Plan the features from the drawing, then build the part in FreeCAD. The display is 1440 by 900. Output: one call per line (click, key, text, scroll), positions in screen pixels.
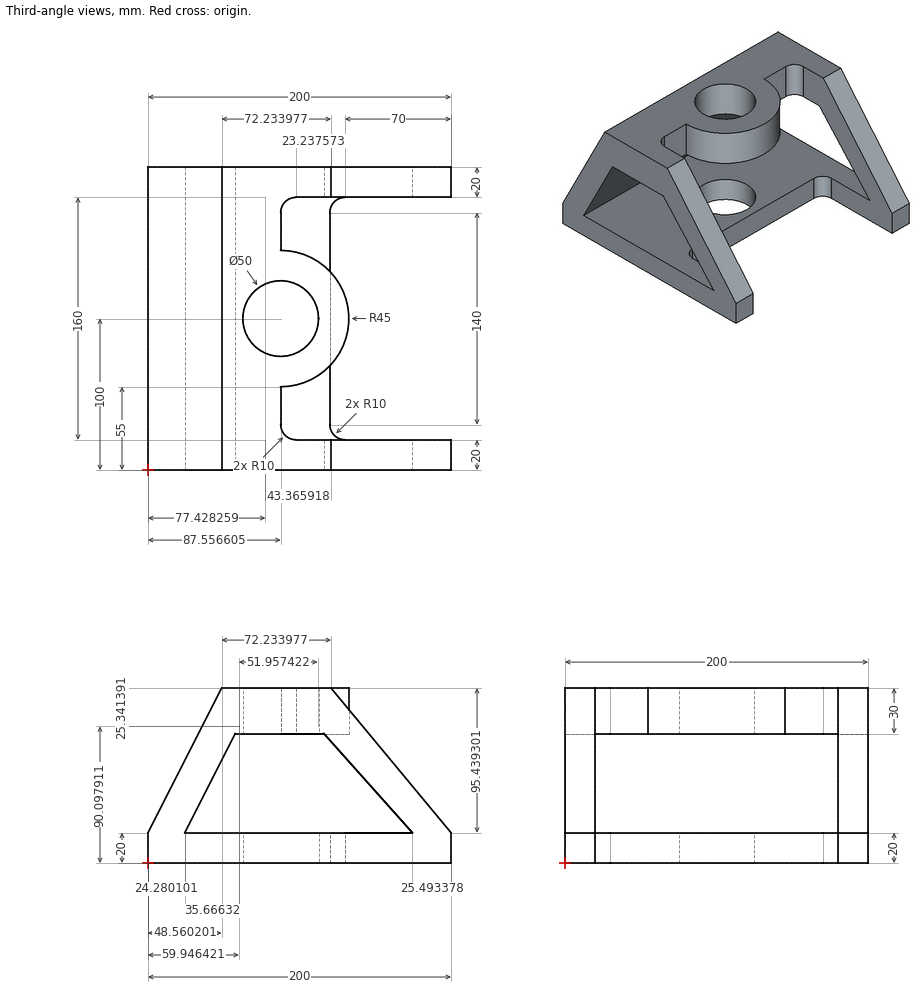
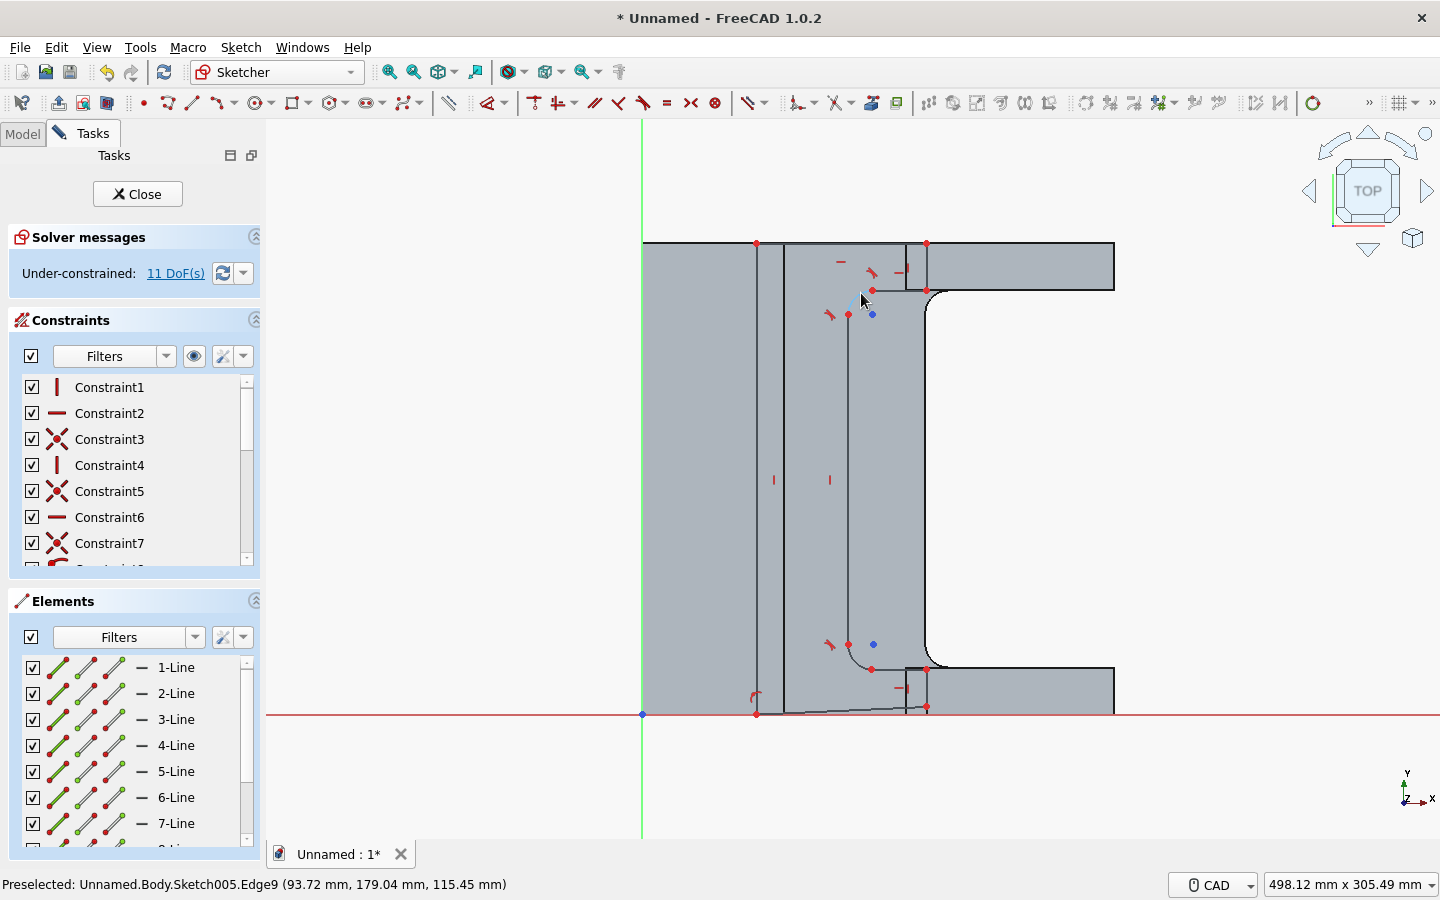
click(910, 670)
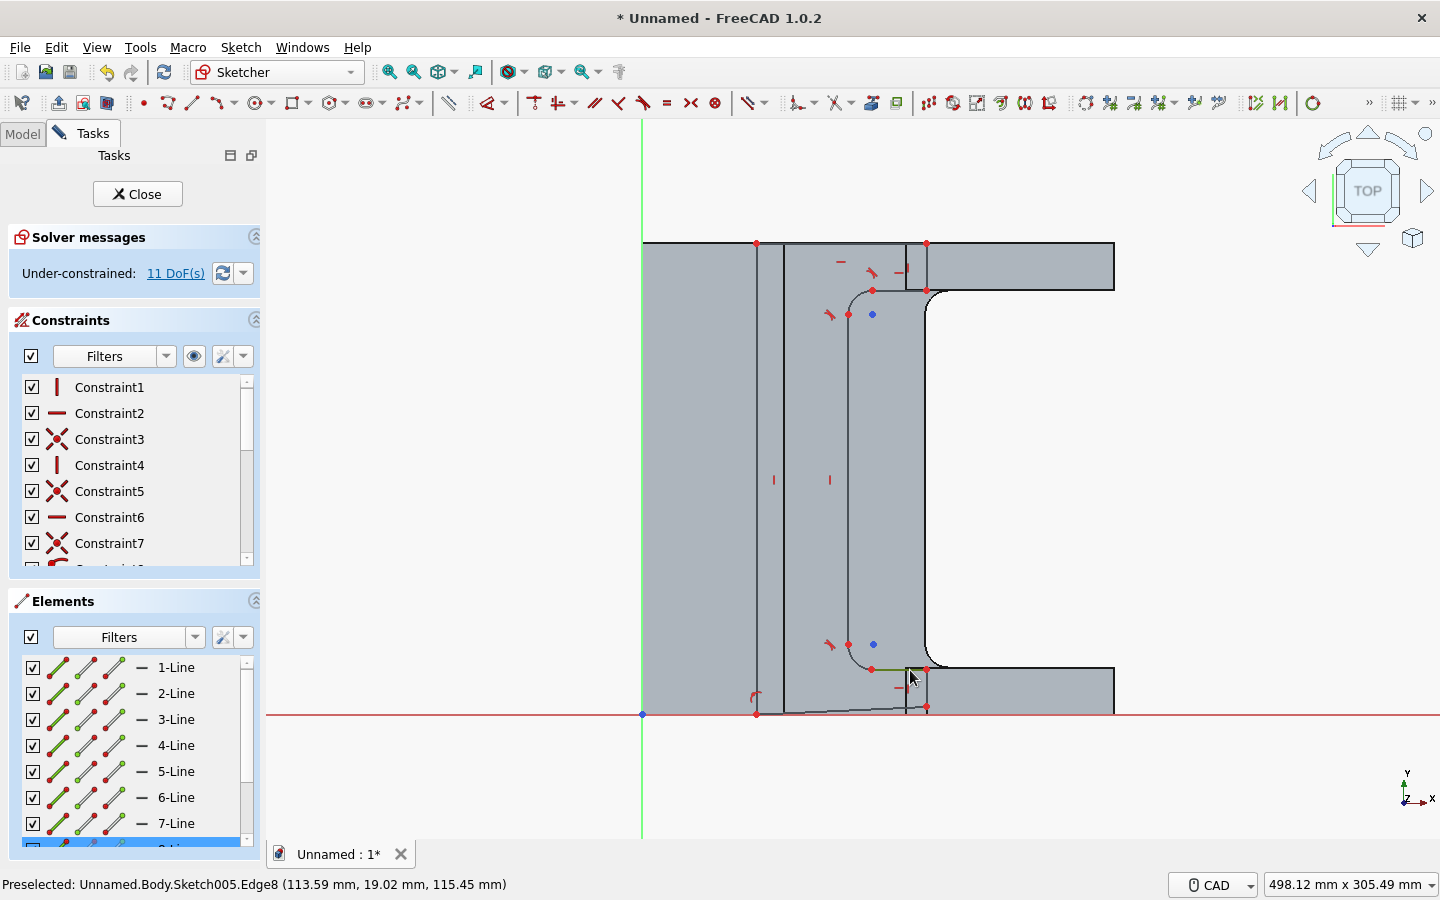
click(851, 655)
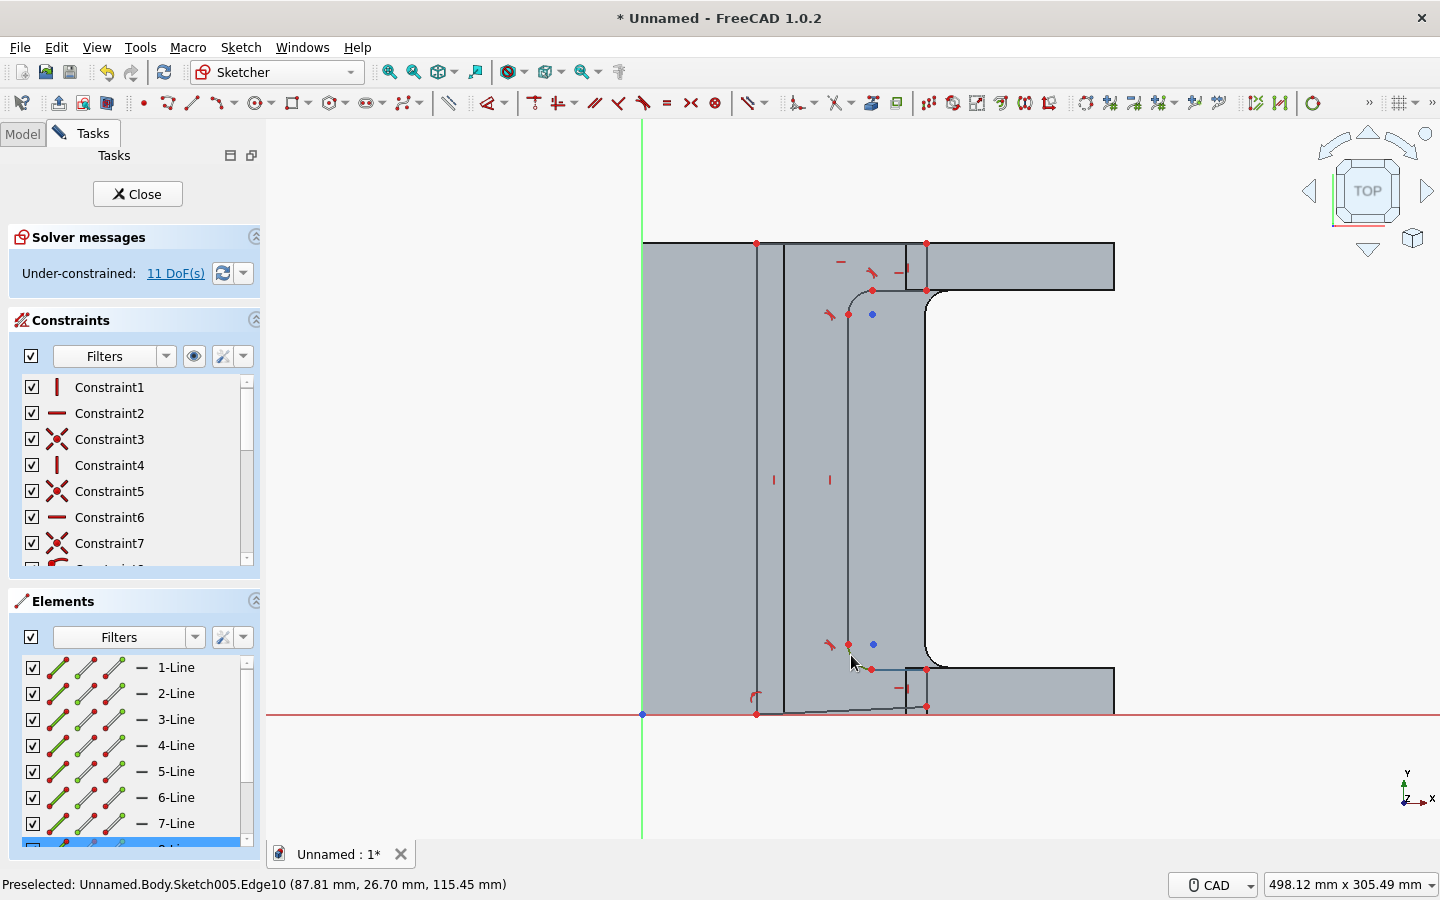
key(t)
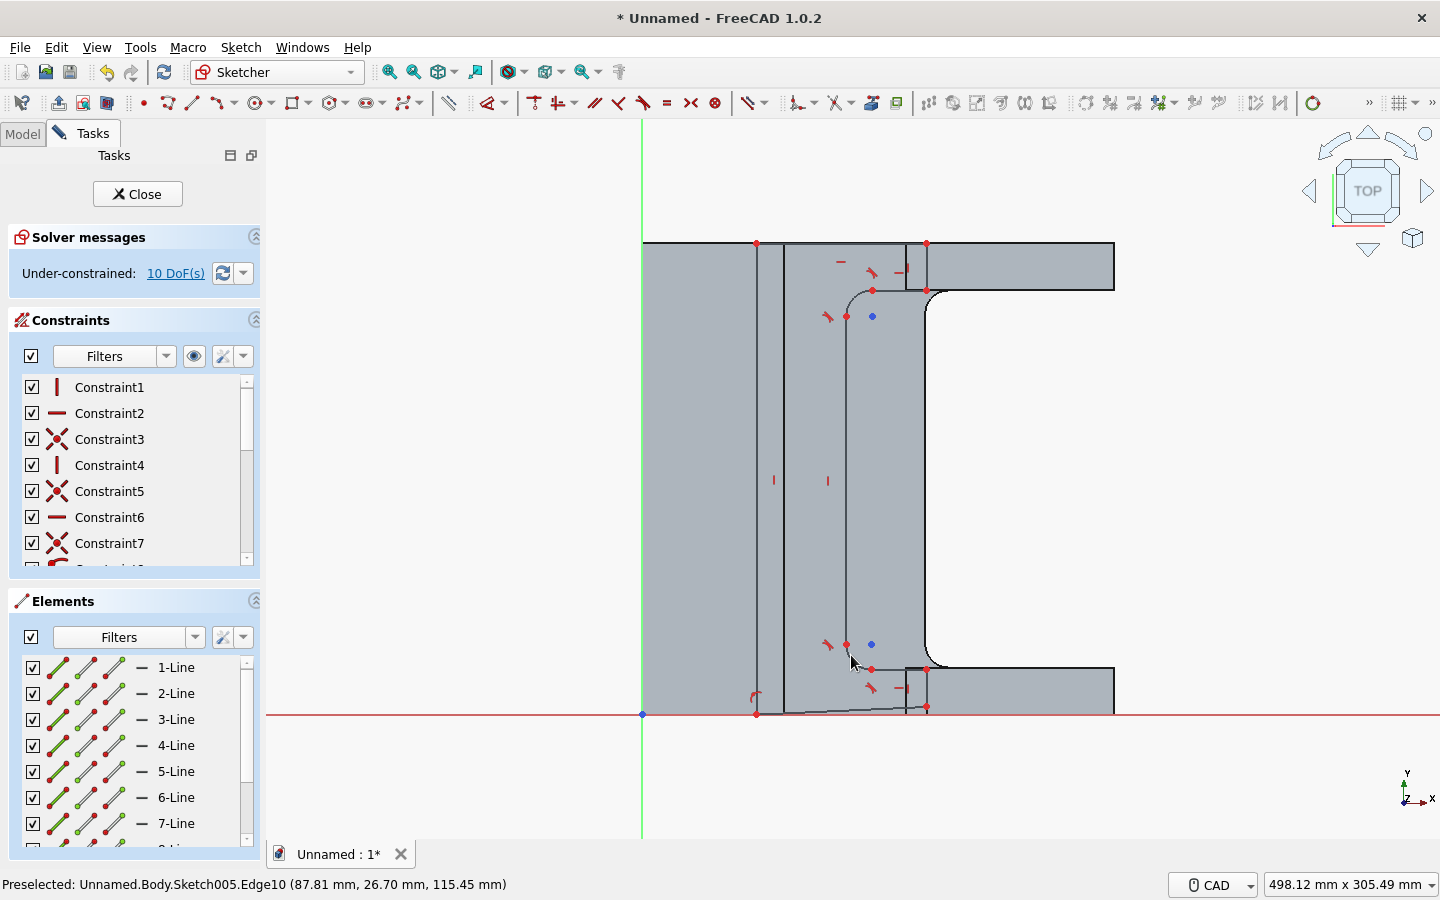
click(808, 712)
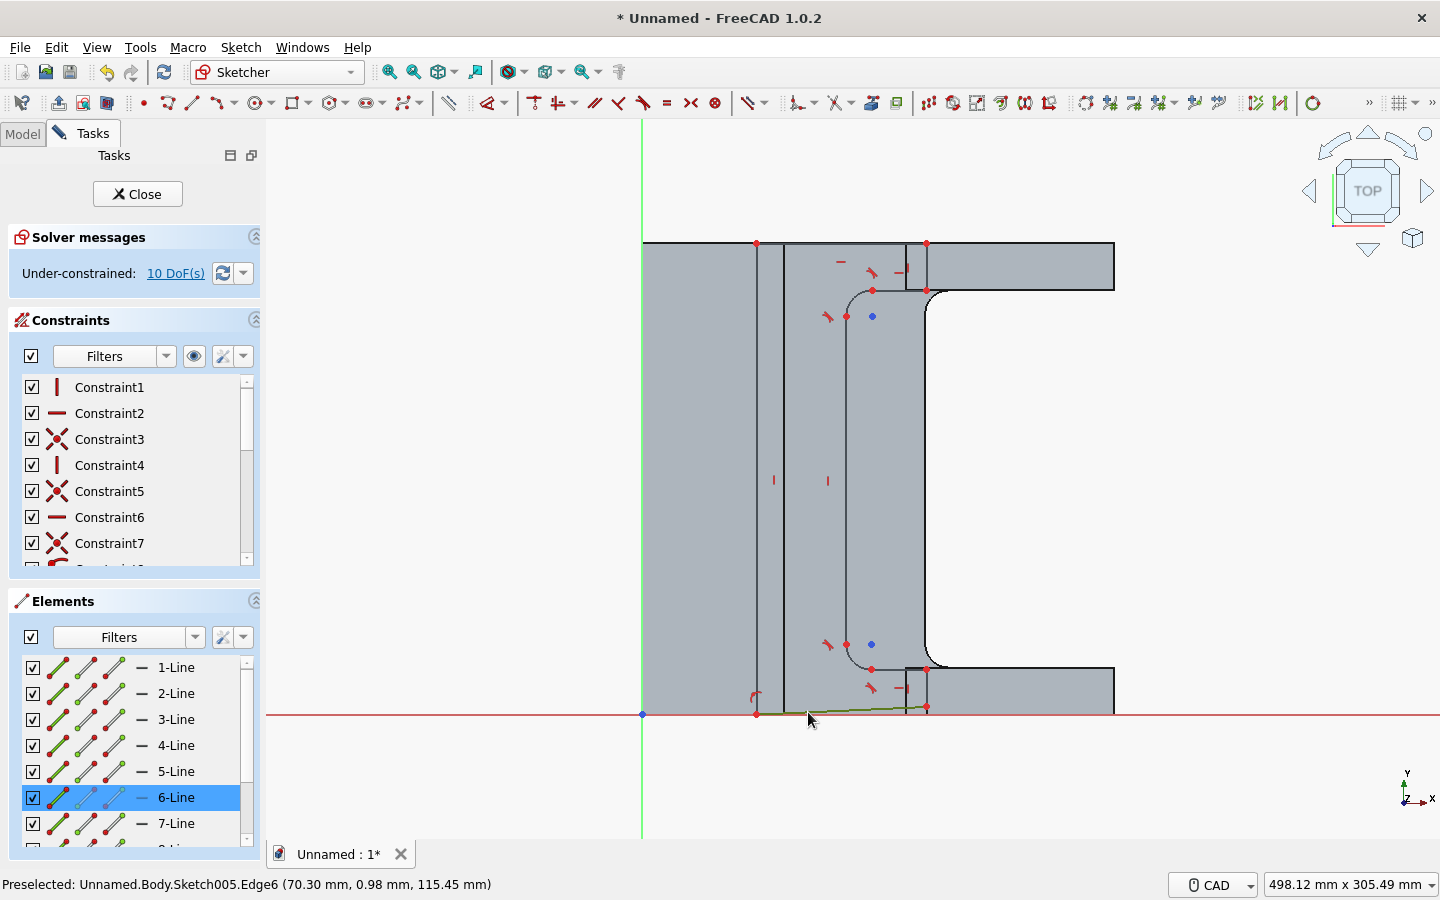
key(h)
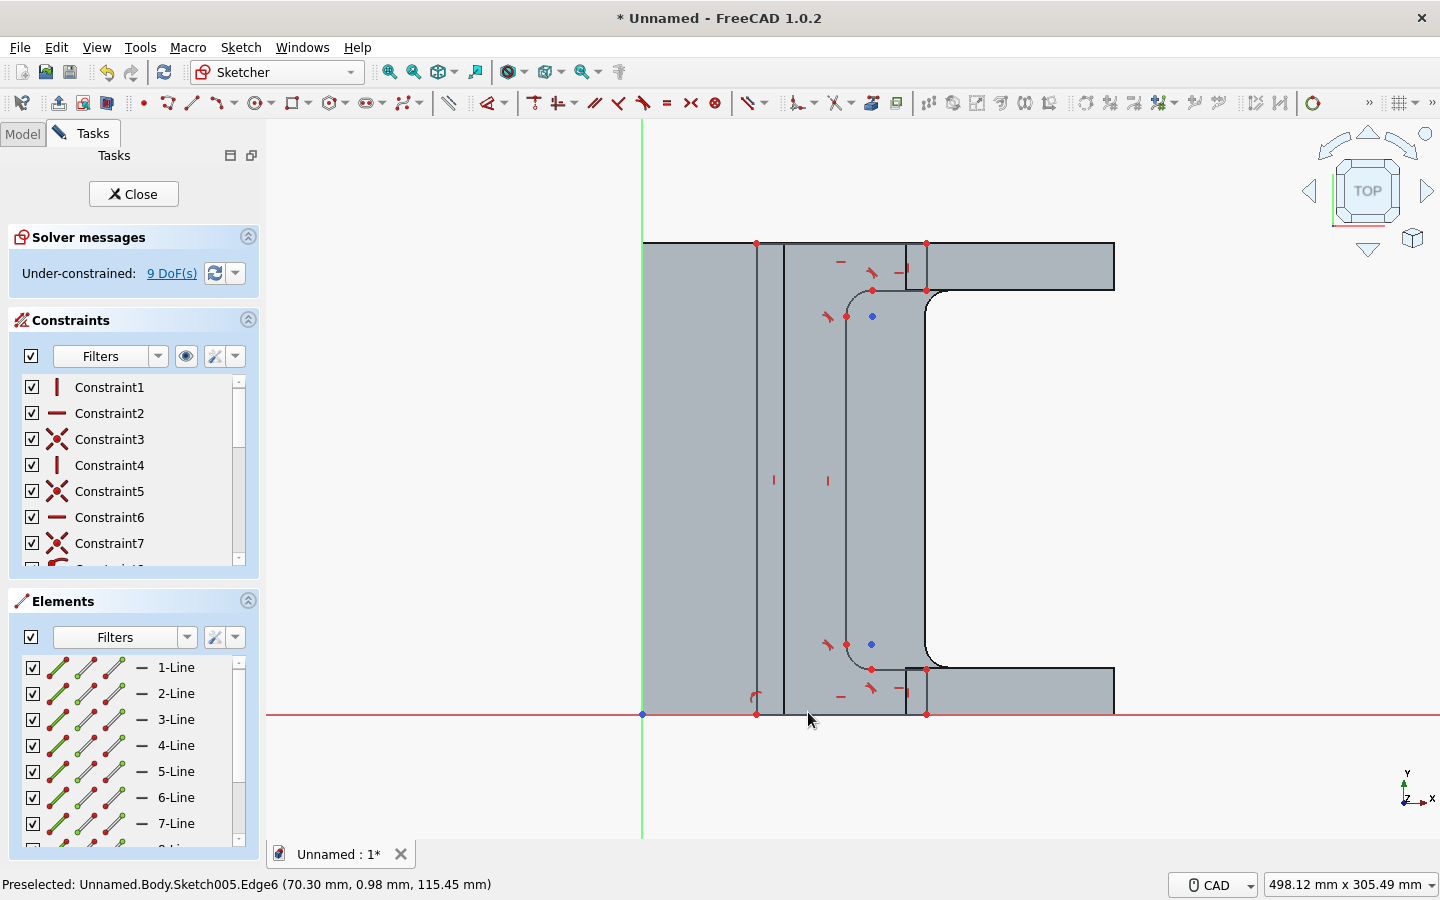
click(860, 293)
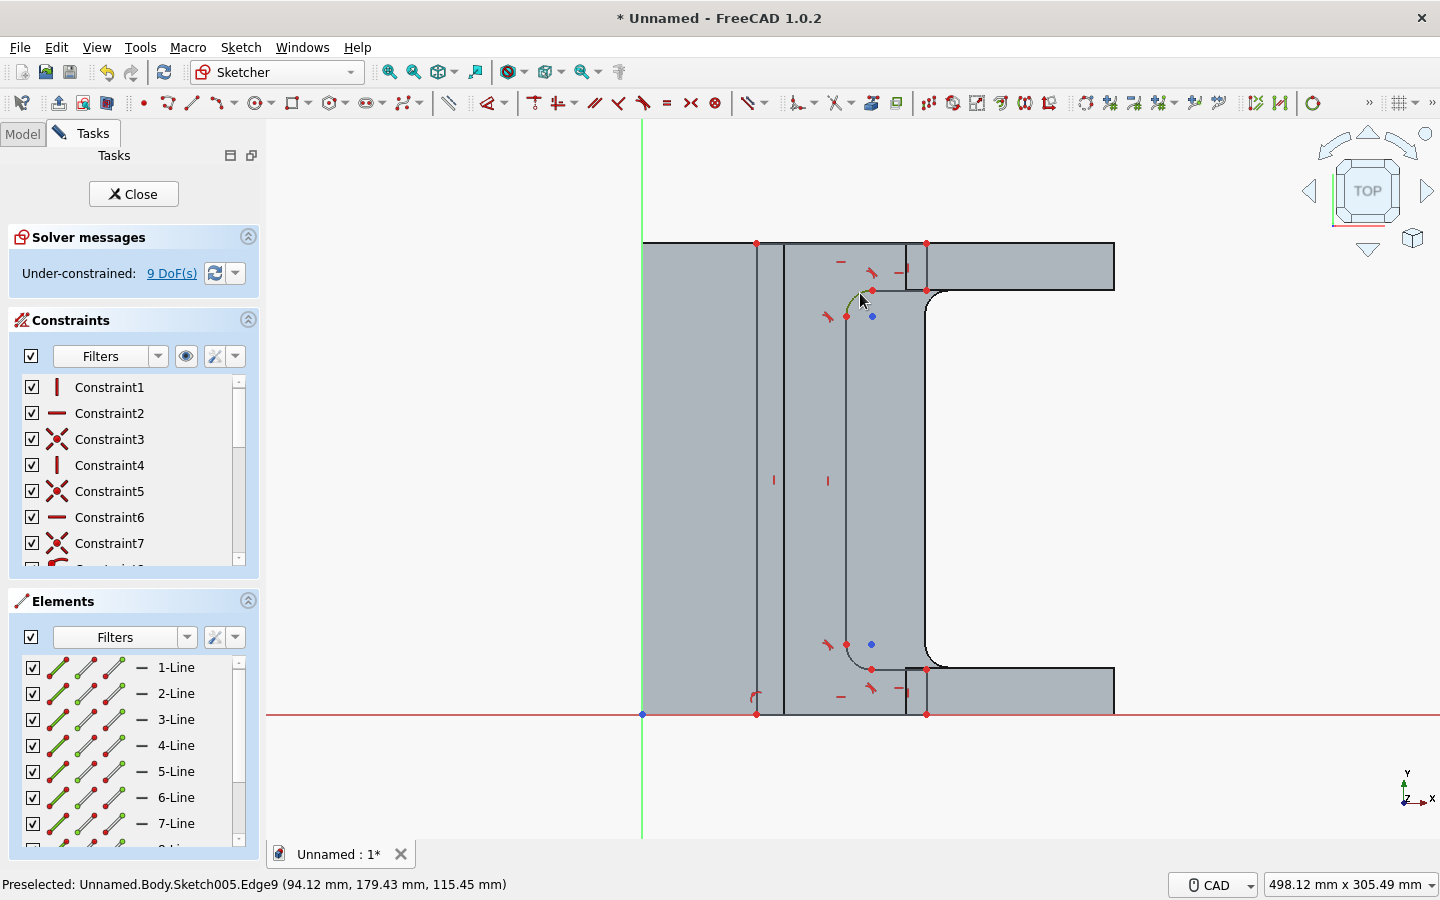
click(849, 656)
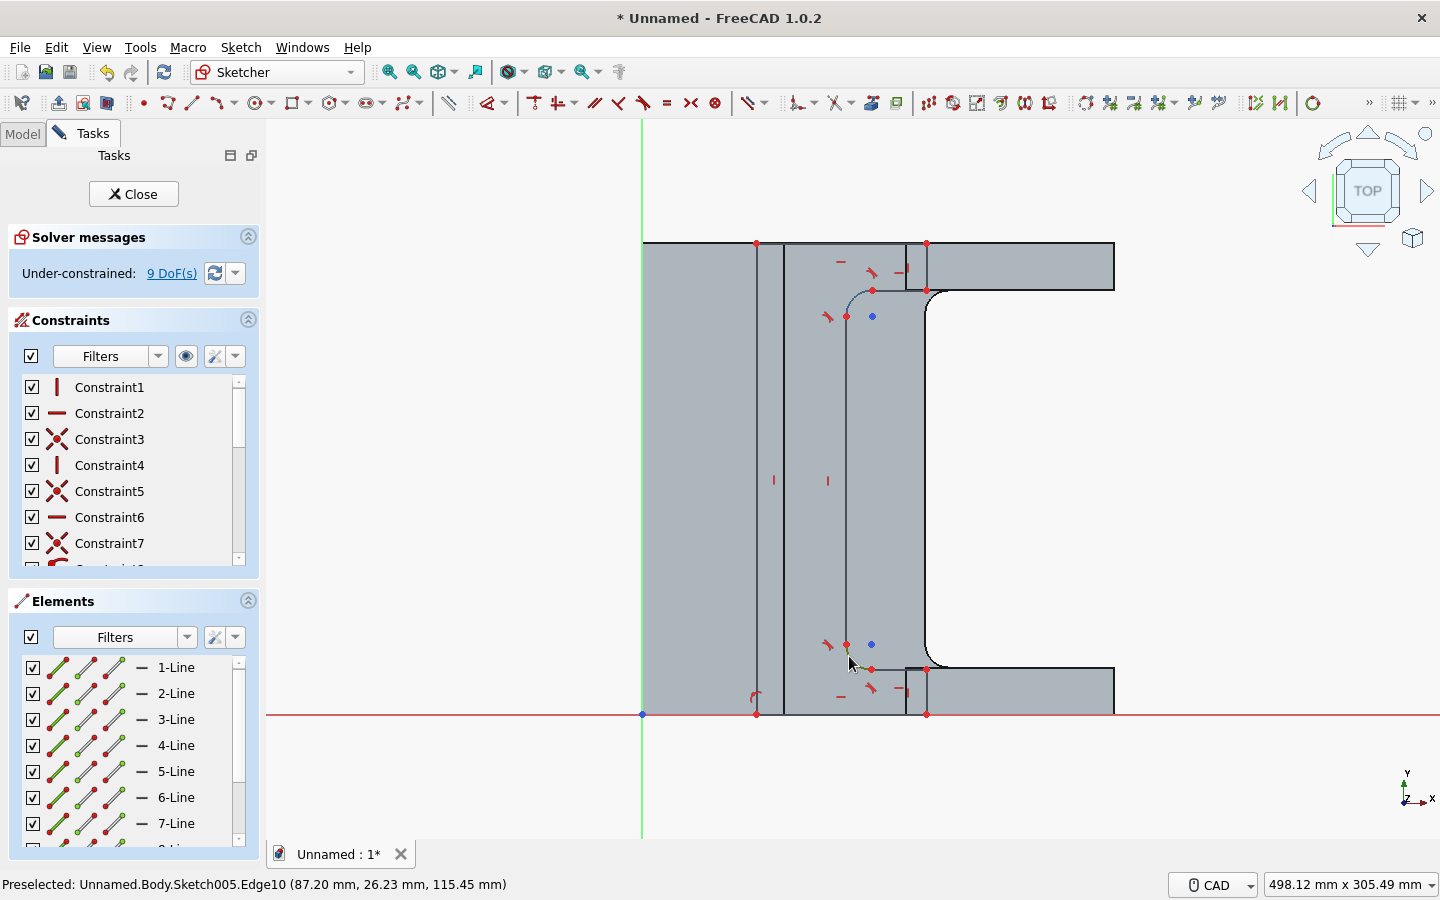
click(668, 104)